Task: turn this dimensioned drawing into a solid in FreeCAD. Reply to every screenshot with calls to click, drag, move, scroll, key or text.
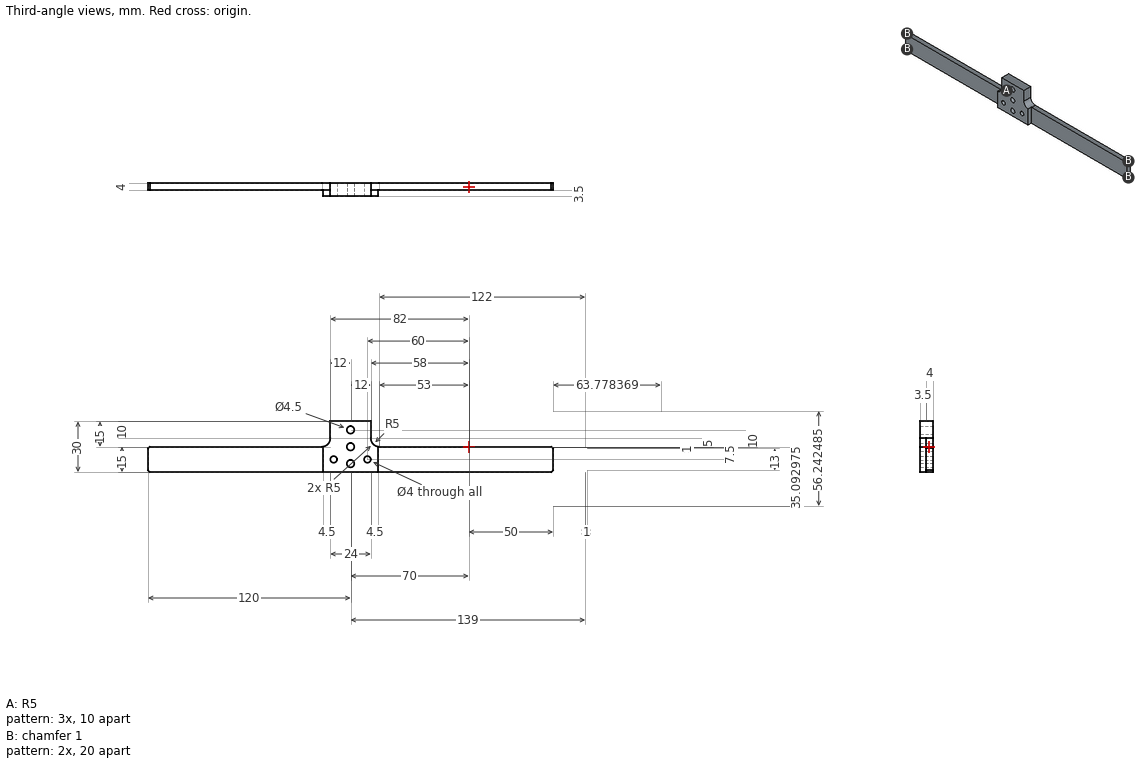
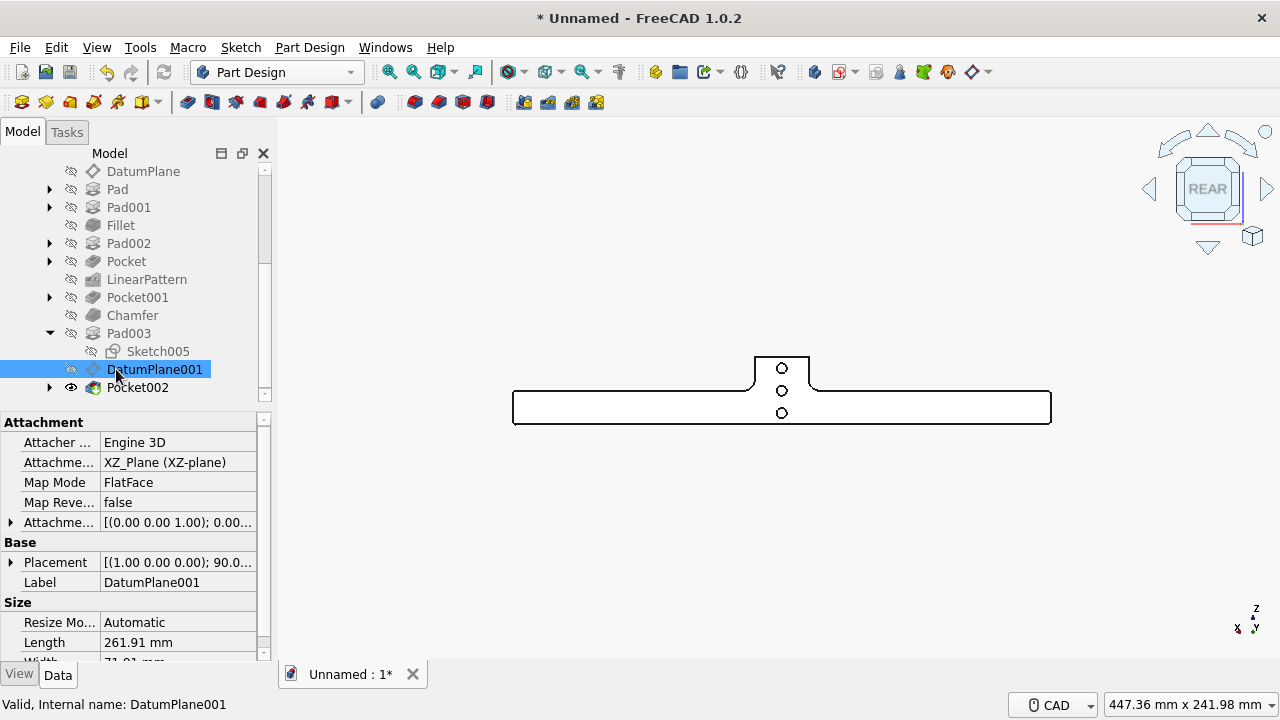
click(551, 409)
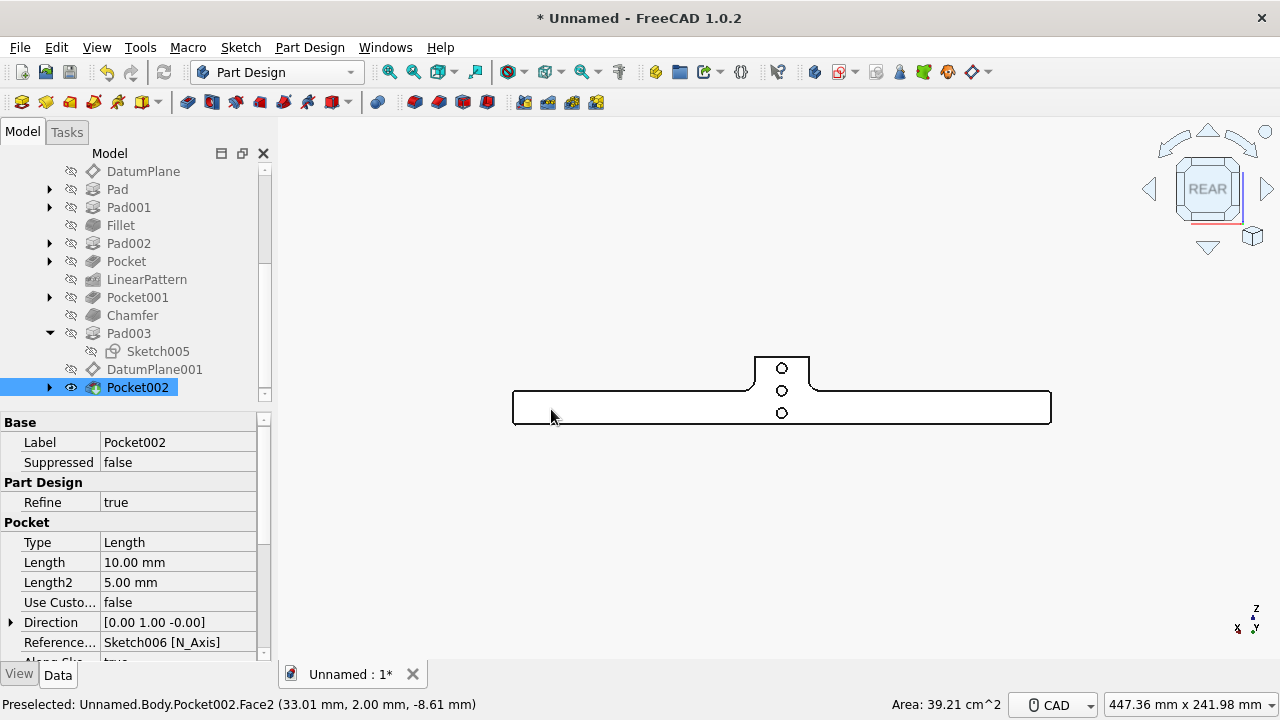
click(840, 72)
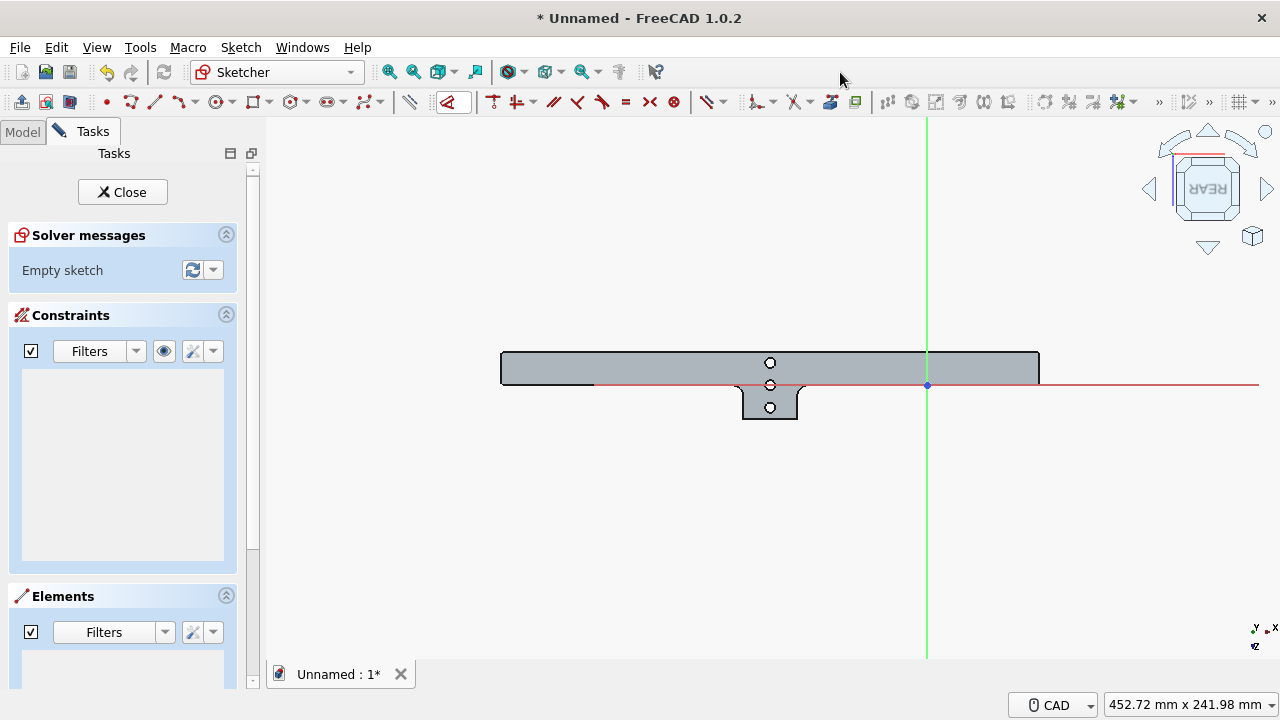
scroll(797, 367, up, 15)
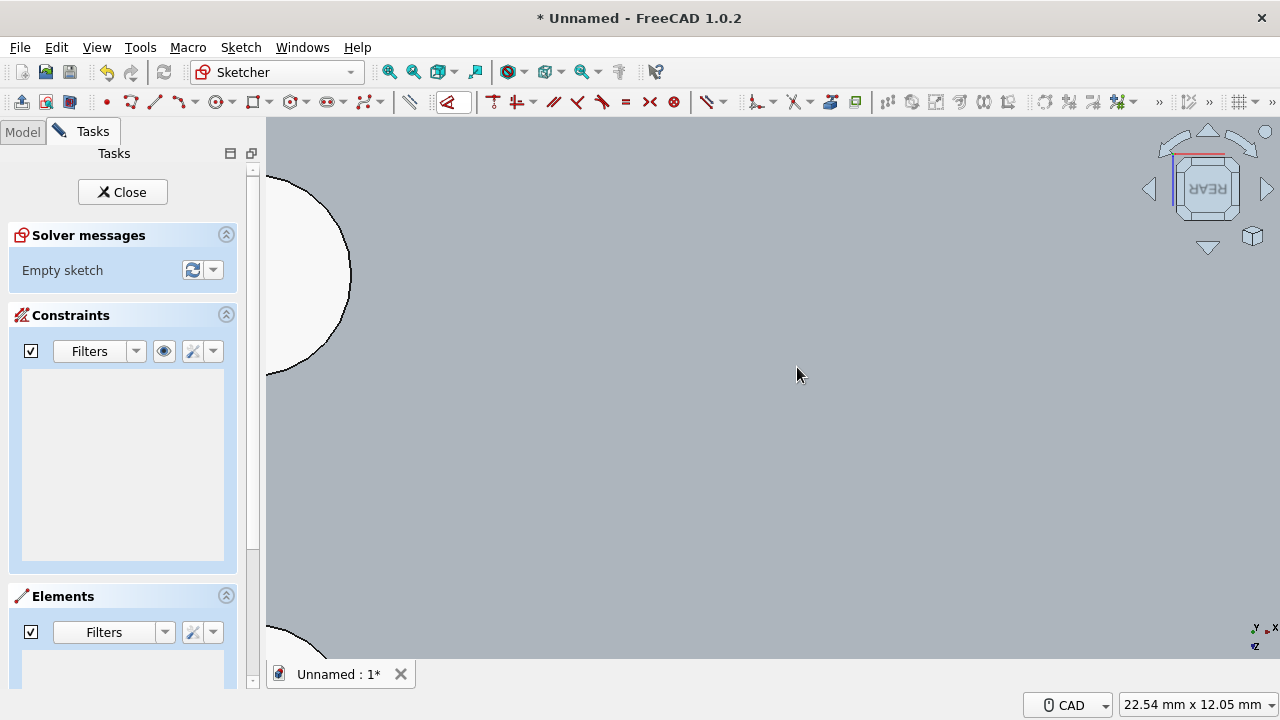
scroll(695, 388, up, 3)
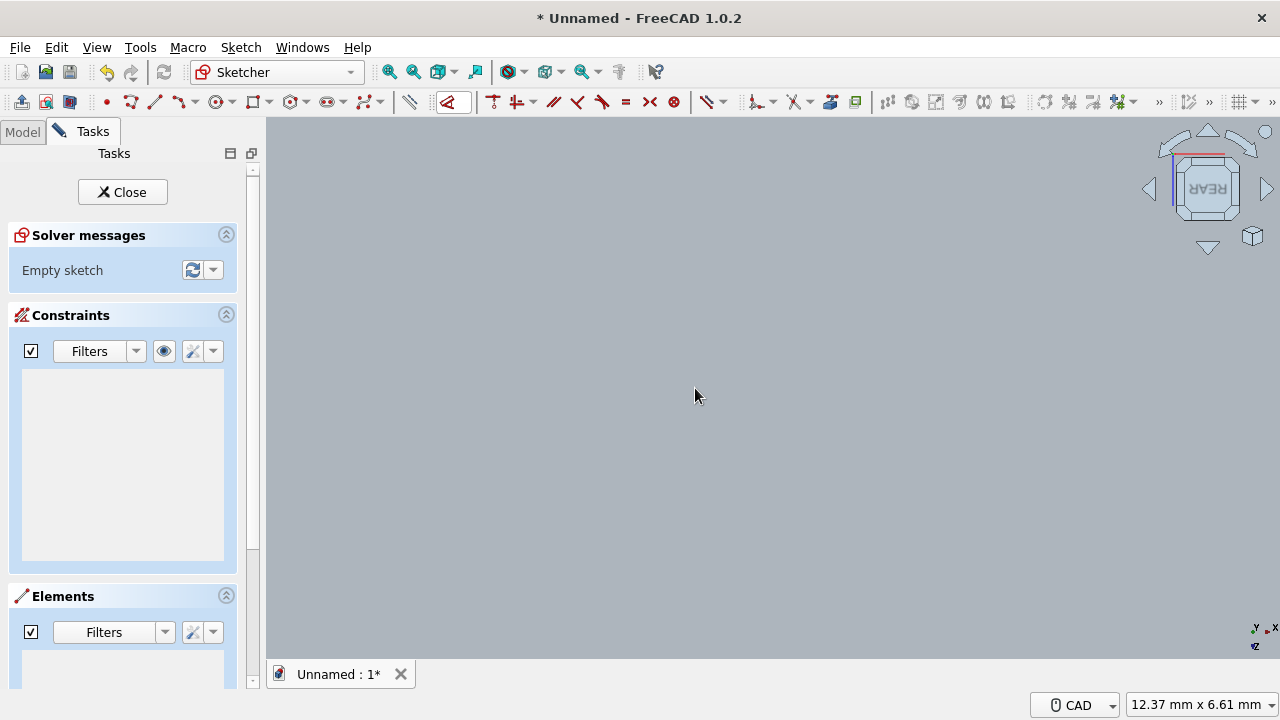
click(216, 102)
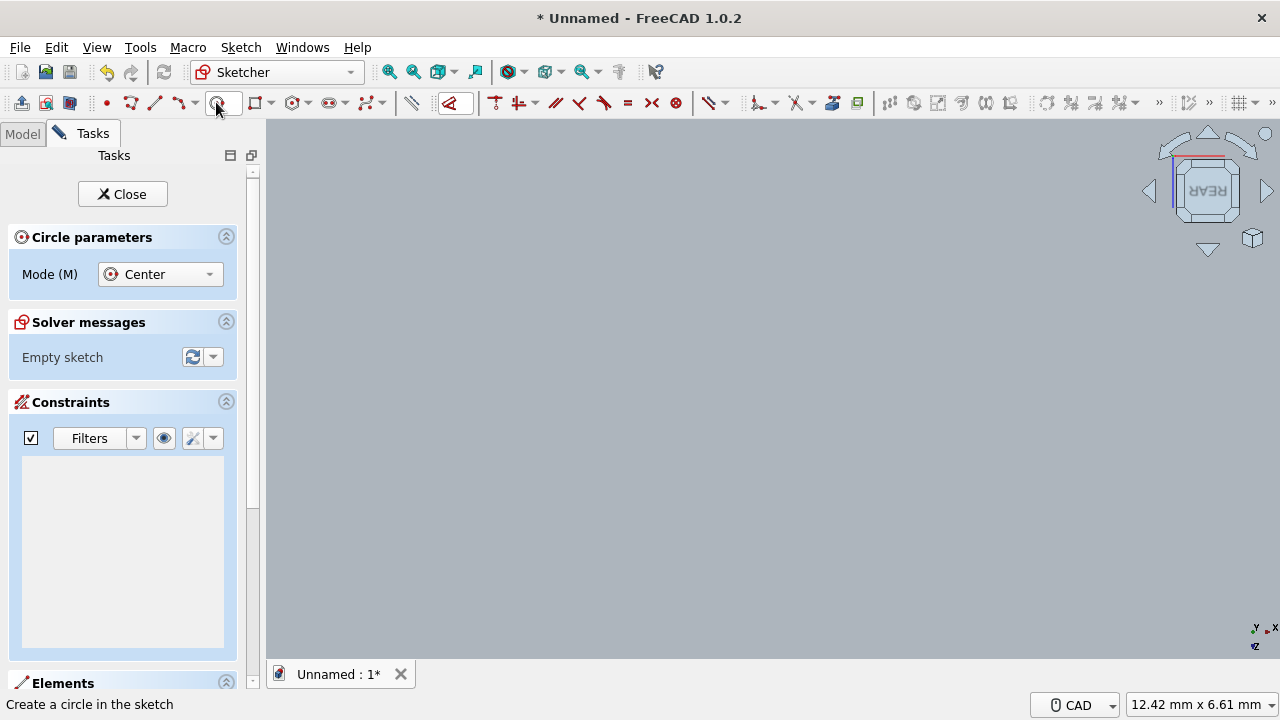
click(704, 388)
click(820, 273)
key(Escape)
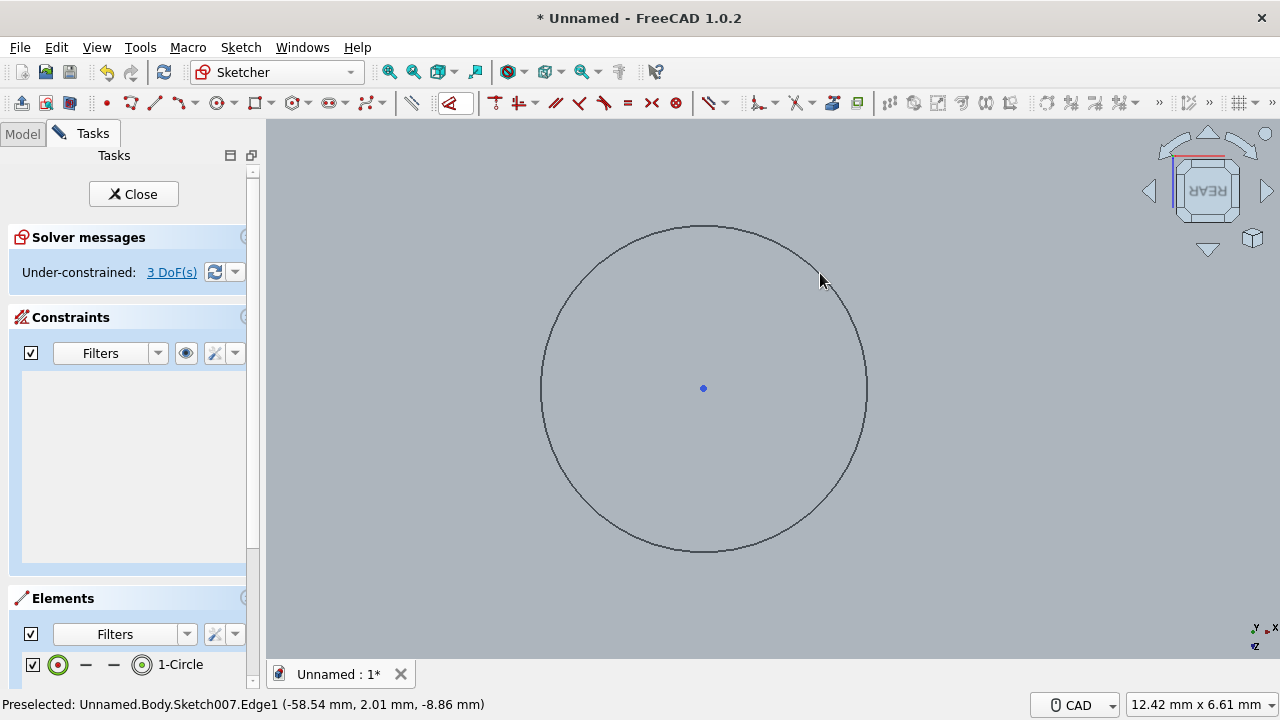
click(819, 273)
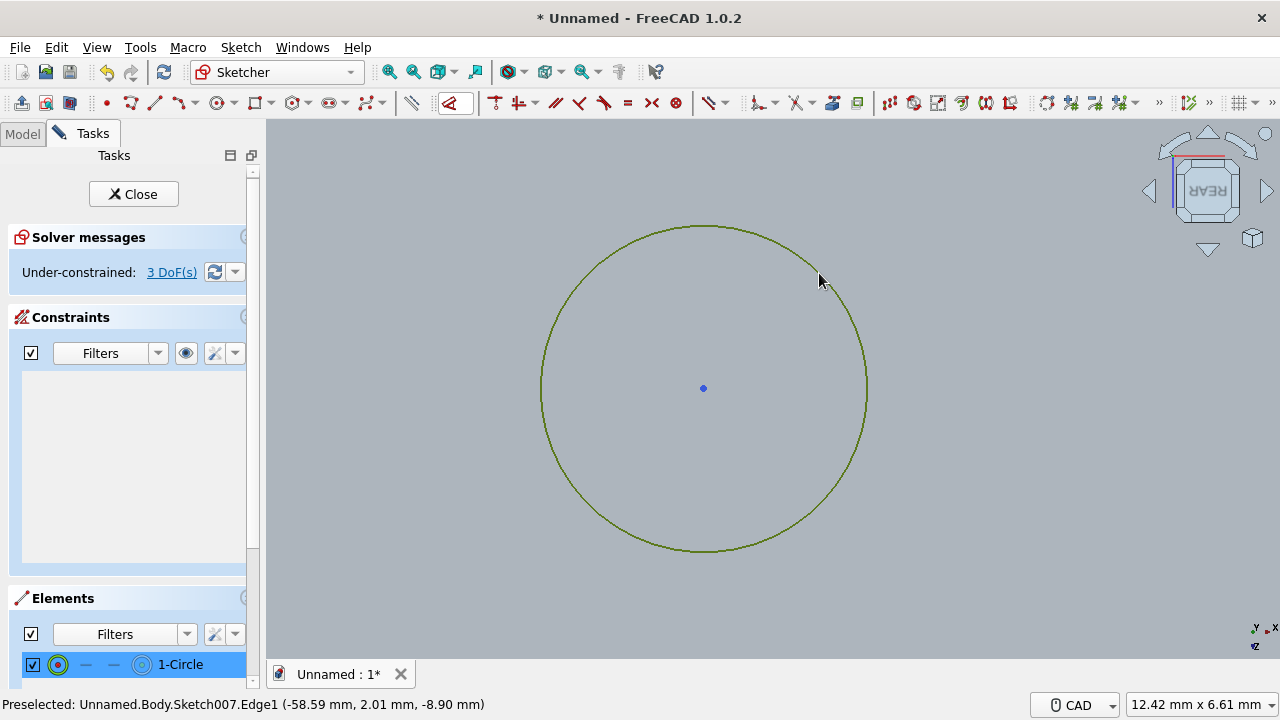
key(k)
key(o)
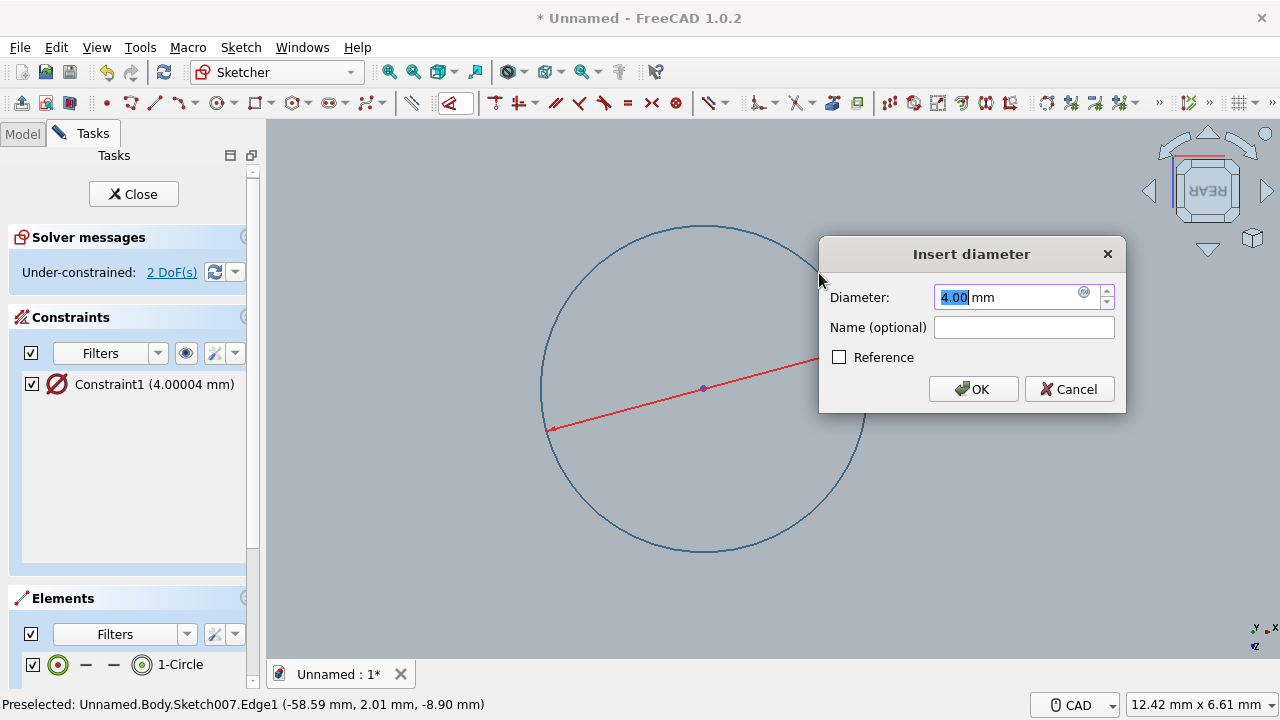
text(4)
key(Return)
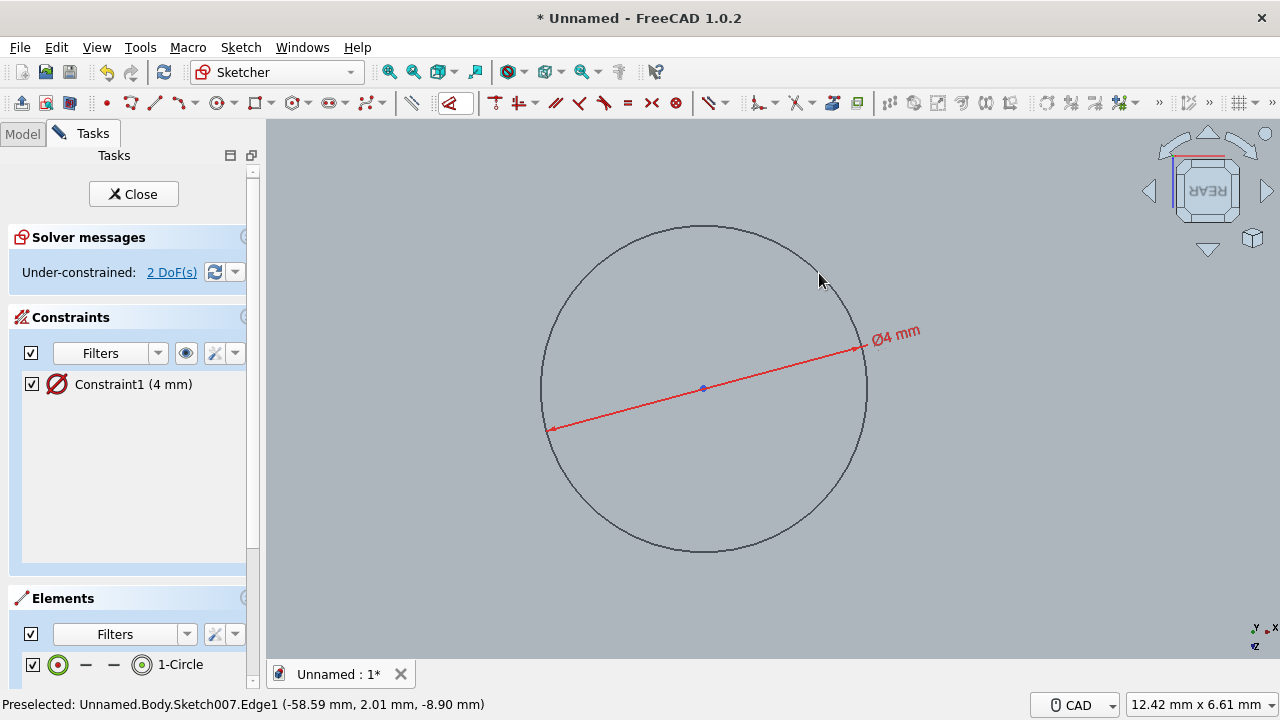
click(704, 389)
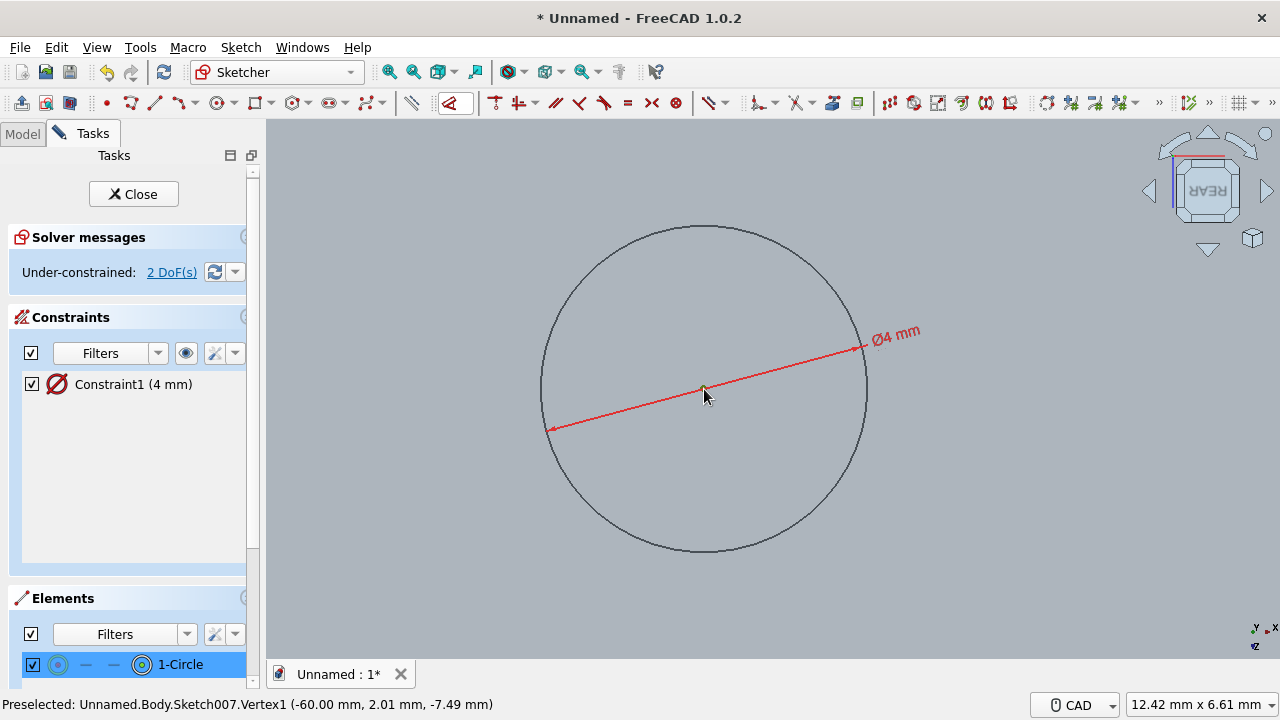
click(468, 104)